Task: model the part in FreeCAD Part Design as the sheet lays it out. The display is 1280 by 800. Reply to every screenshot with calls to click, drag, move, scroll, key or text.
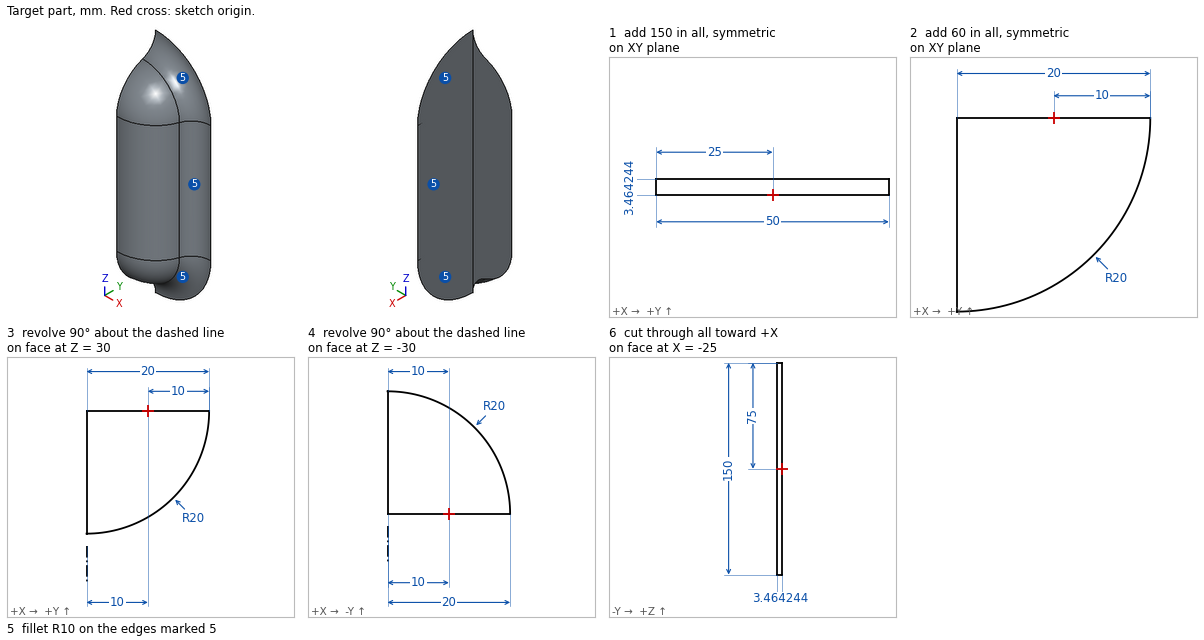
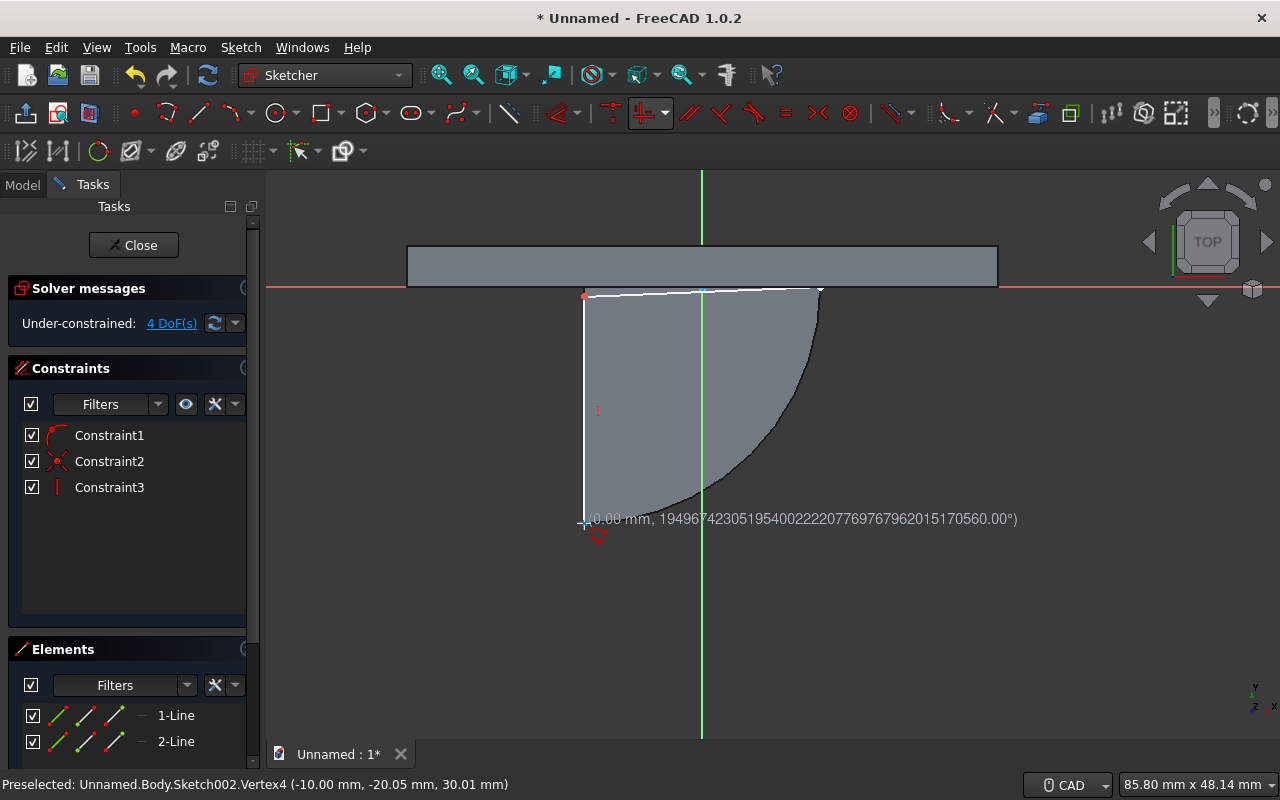
click(232, 114)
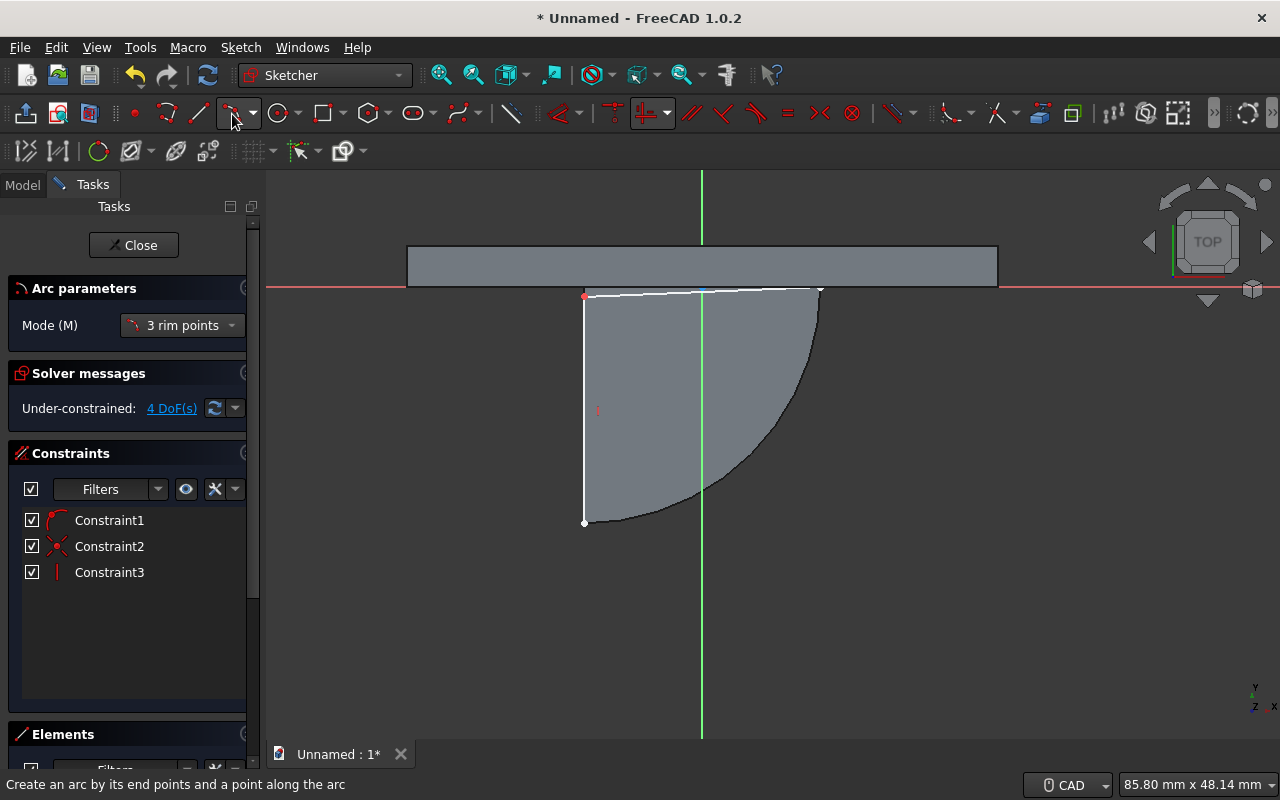
click(584, 524)
click(820, 287)
click(751, 454)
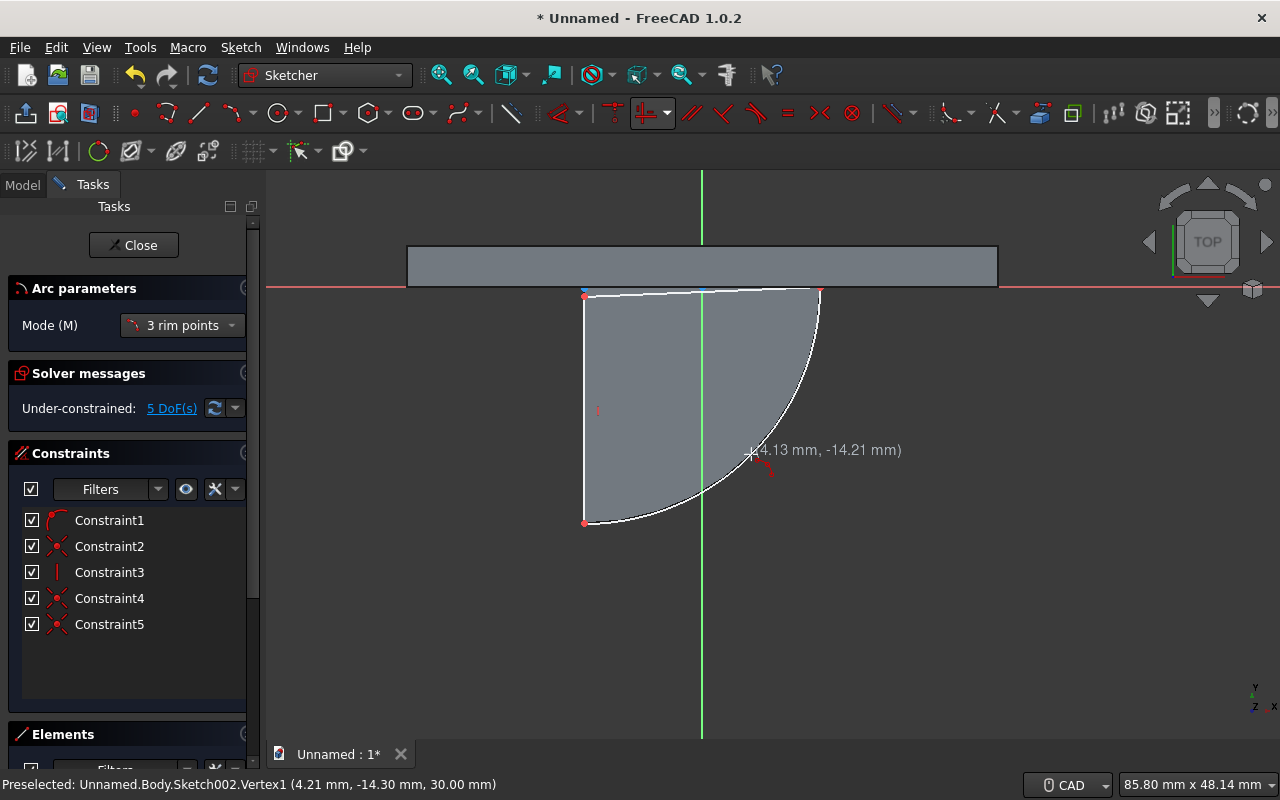
click(200, 114)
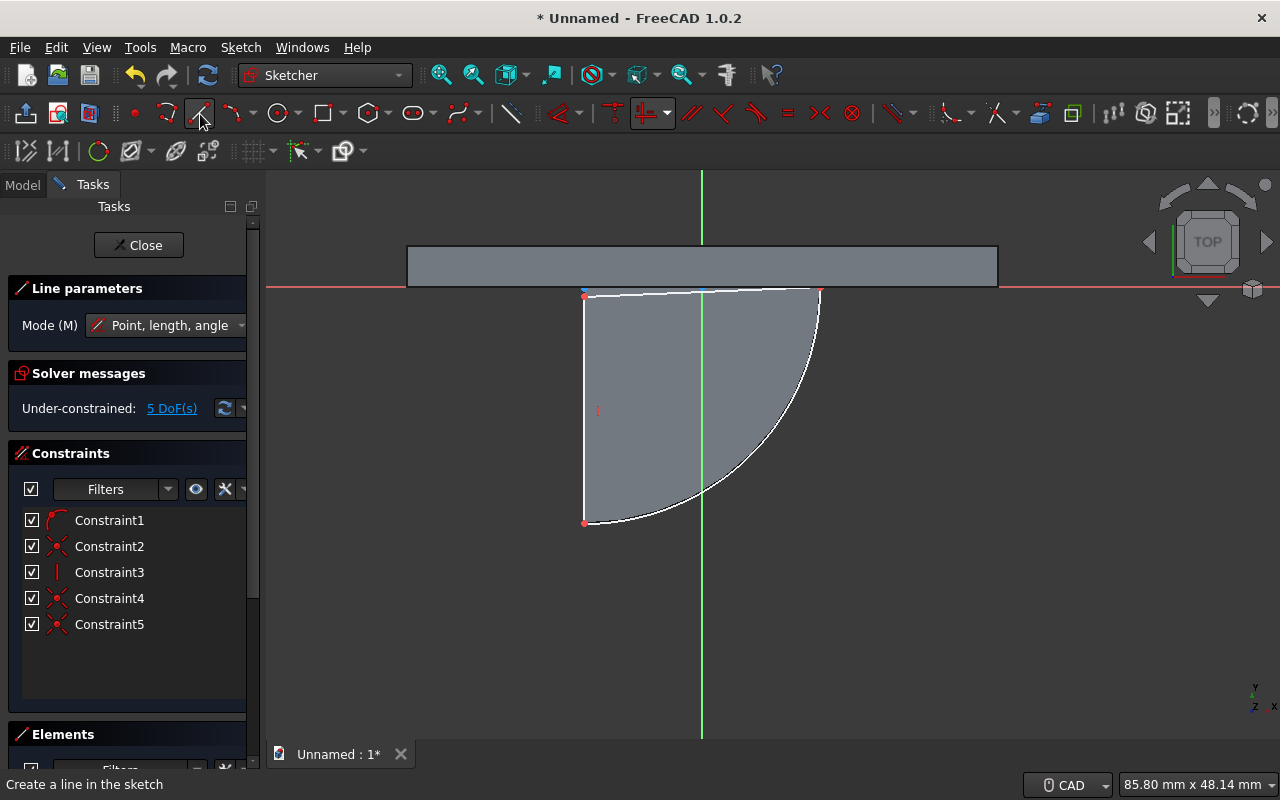
click(584, 547)
click(584, 618)
key(Escape)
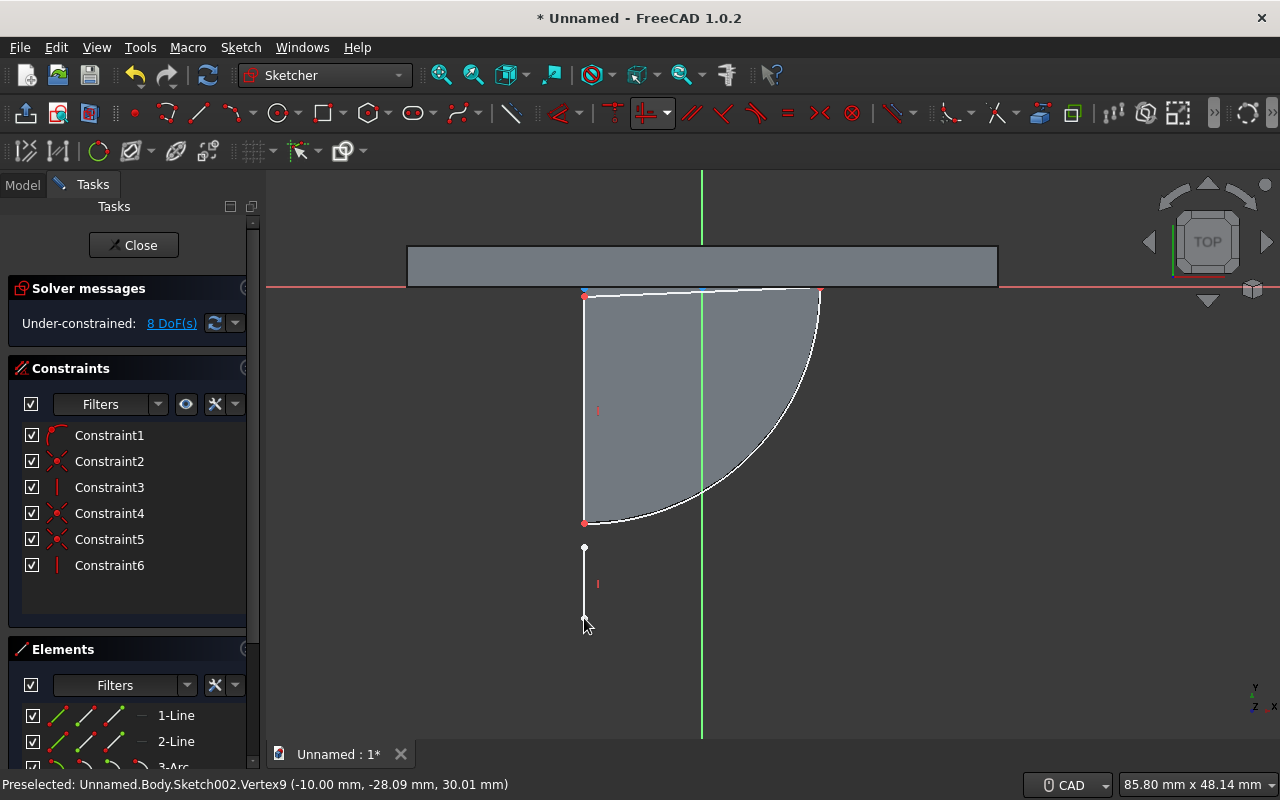
click(584, 569)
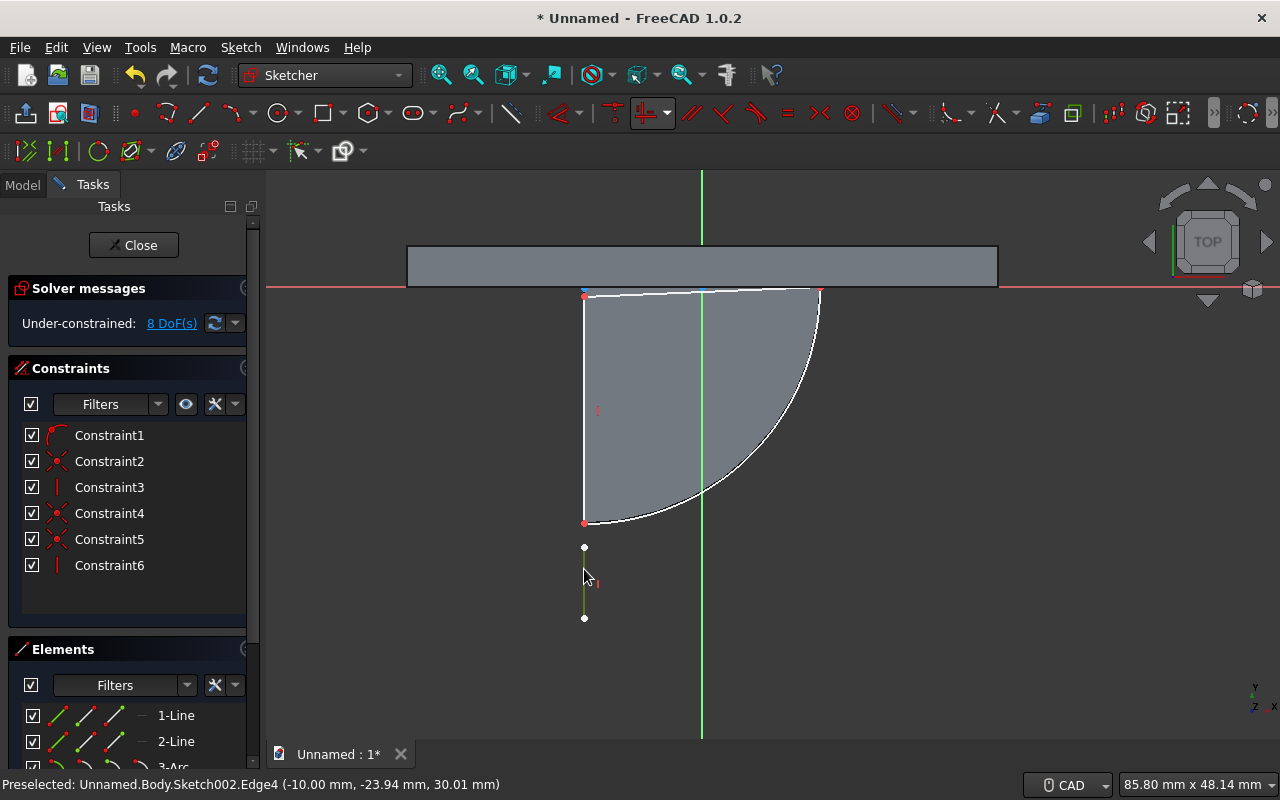
click(512, 114)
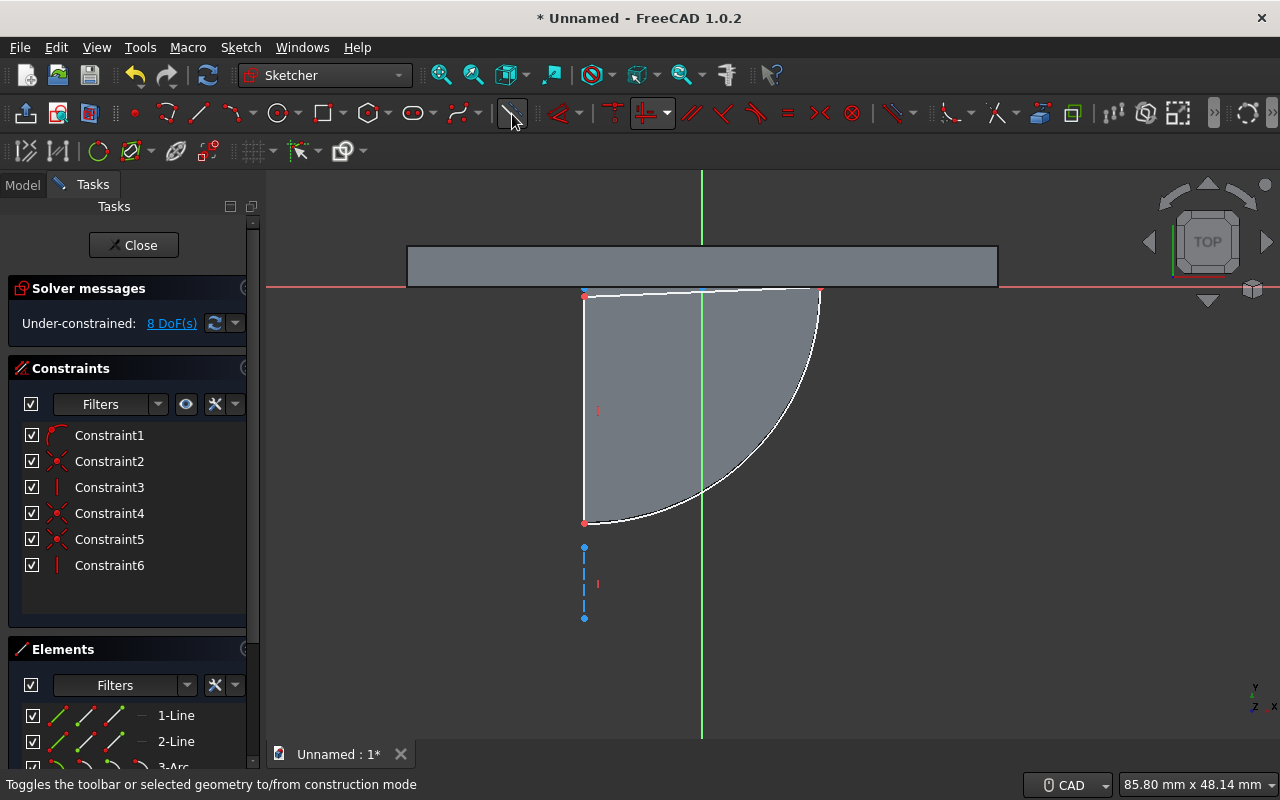
click(749, 290)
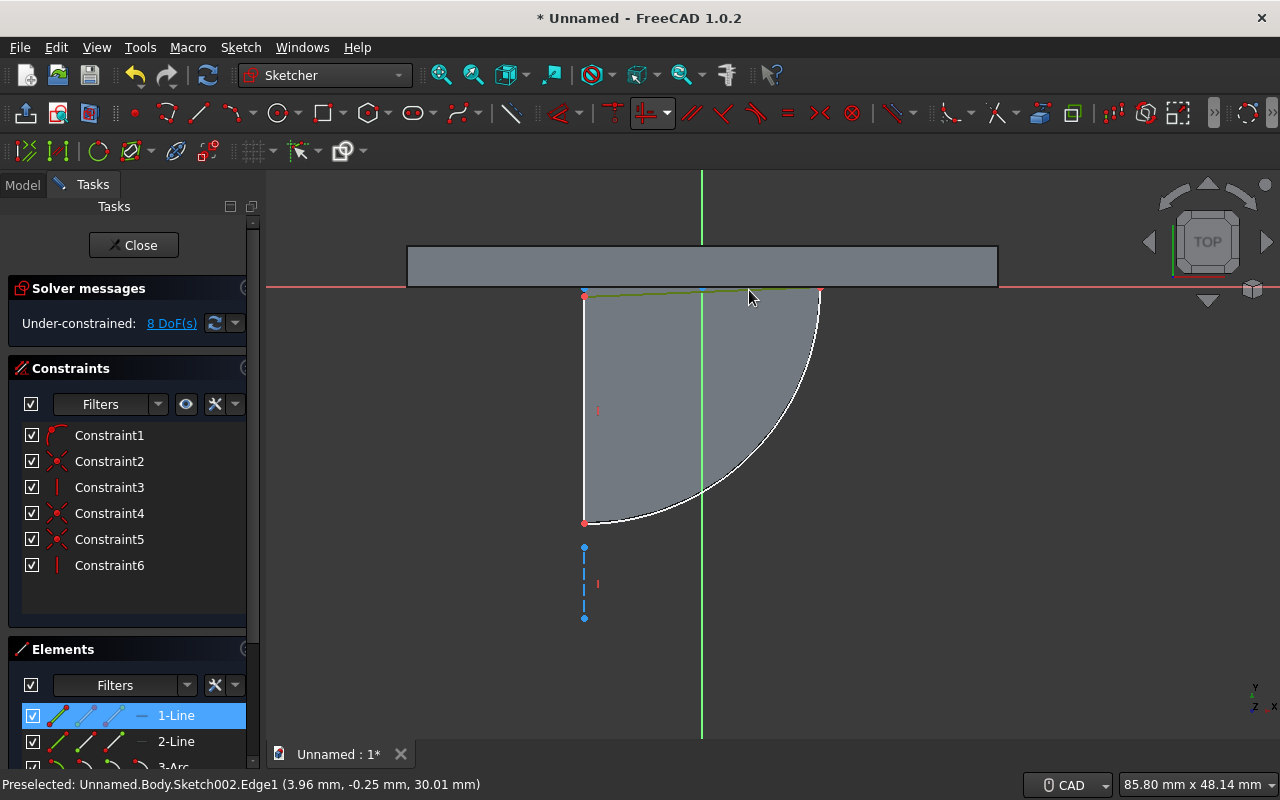
click(670, 114)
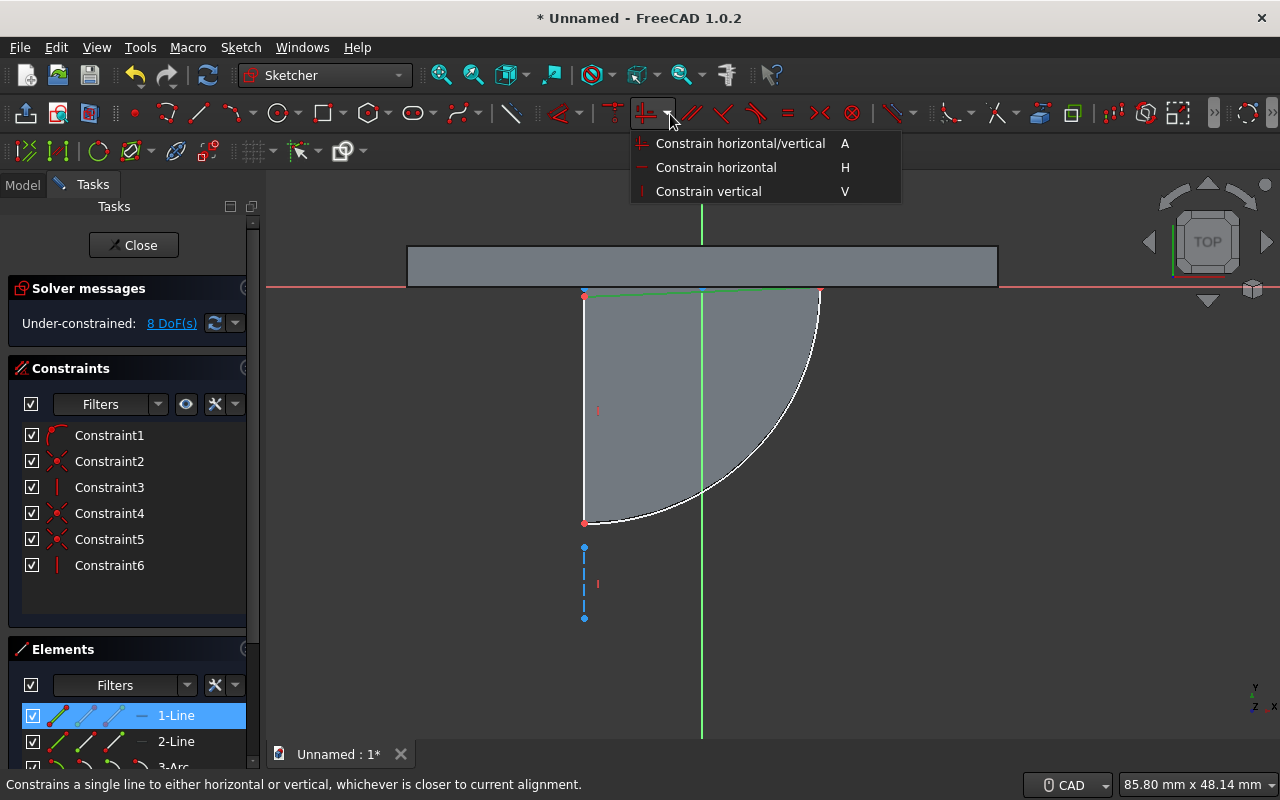
click(766, 167)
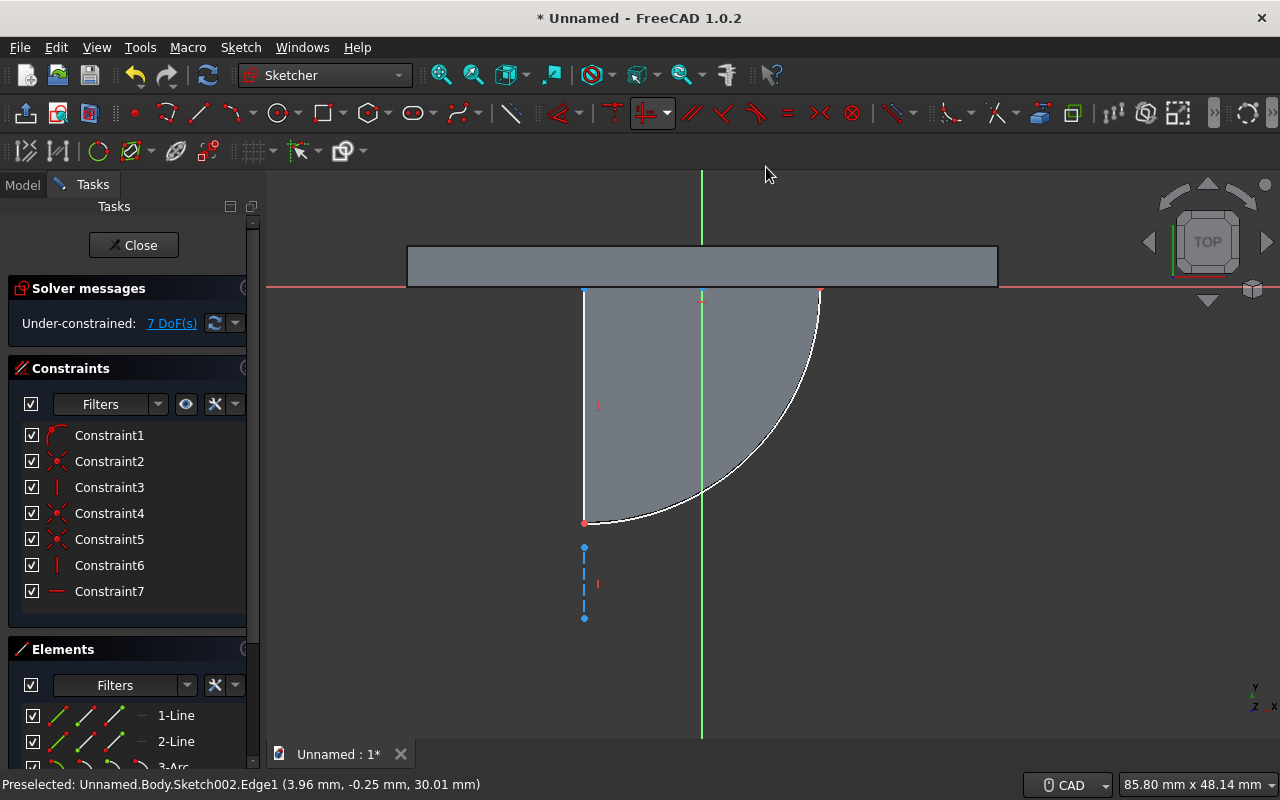
click(584, 288)